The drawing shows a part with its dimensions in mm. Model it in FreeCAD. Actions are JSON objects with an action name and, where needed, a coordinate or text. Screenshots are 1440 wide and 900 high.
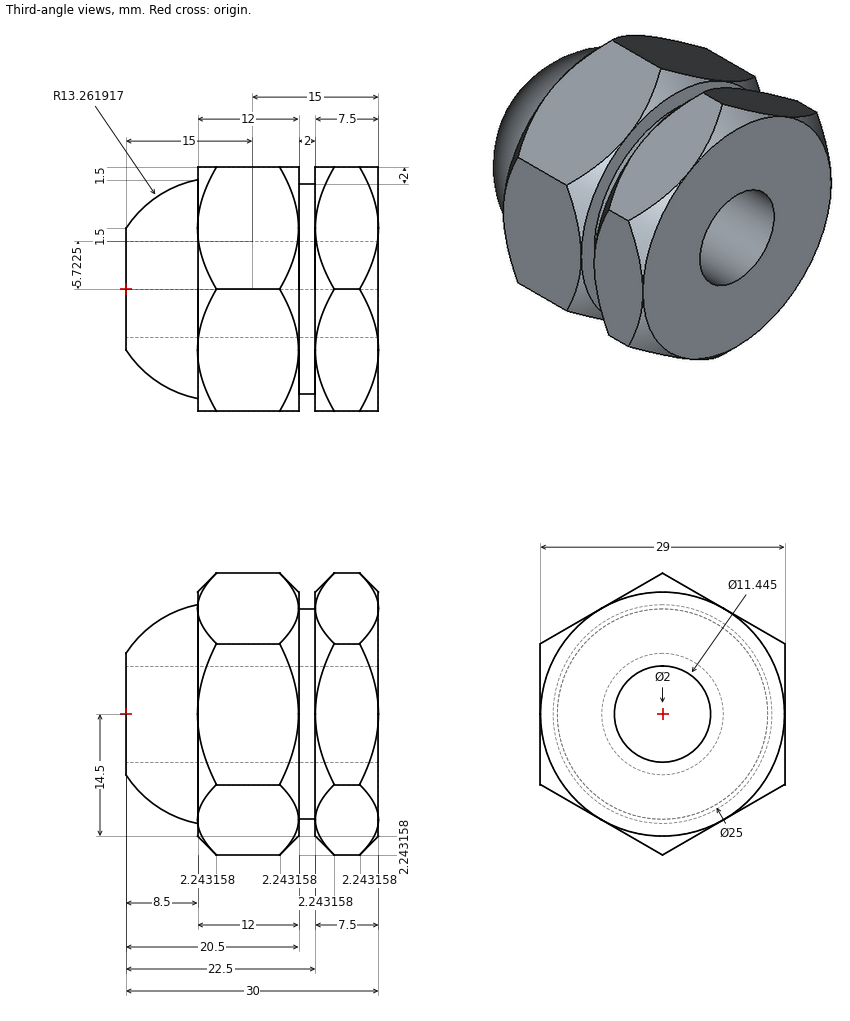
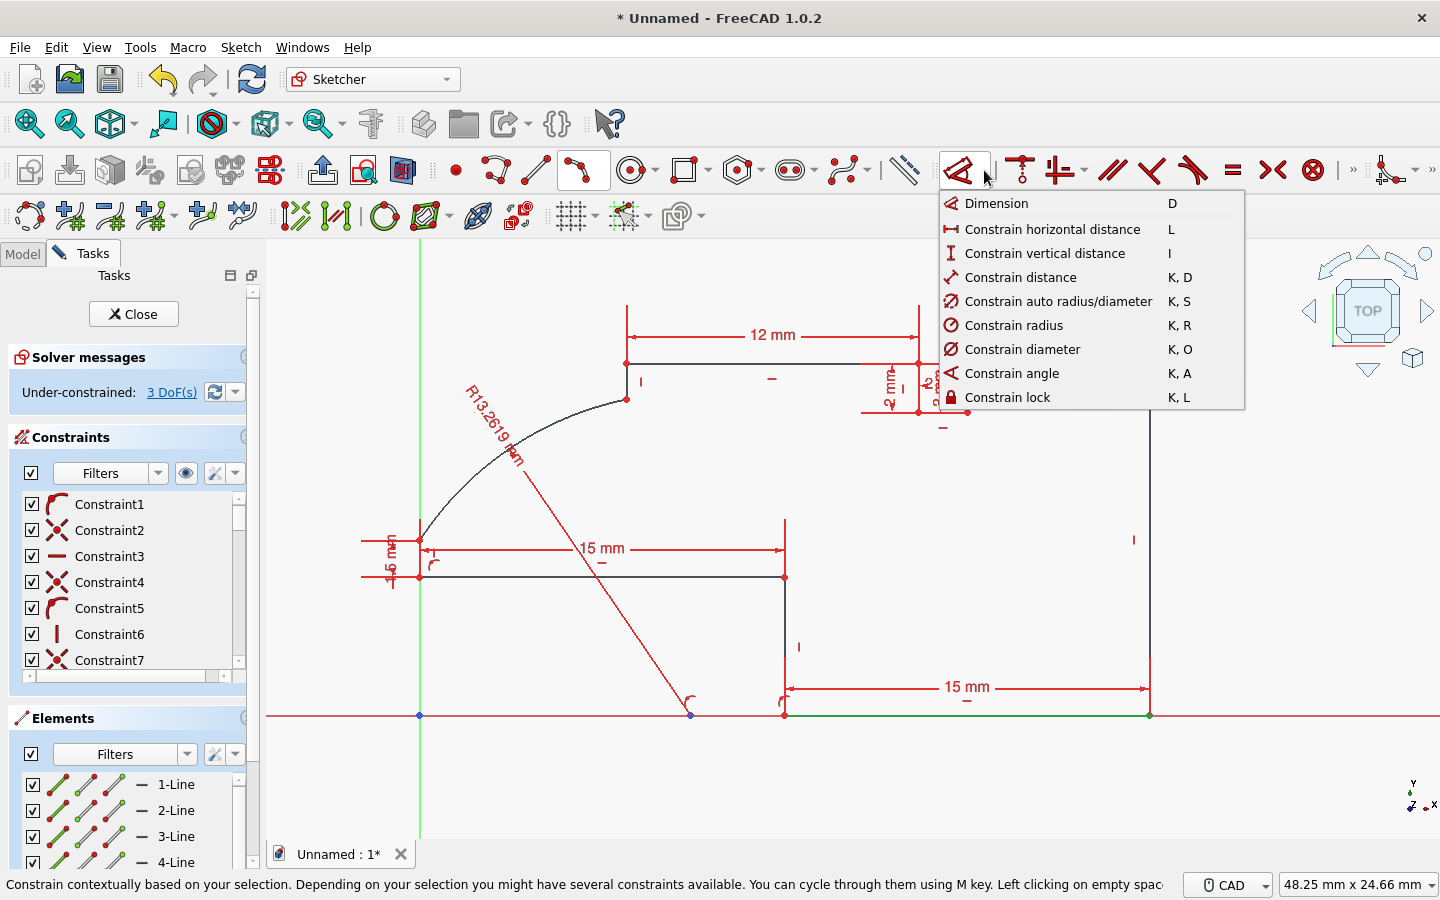
{"action": "left_click", "coordinate": [1092, 229]}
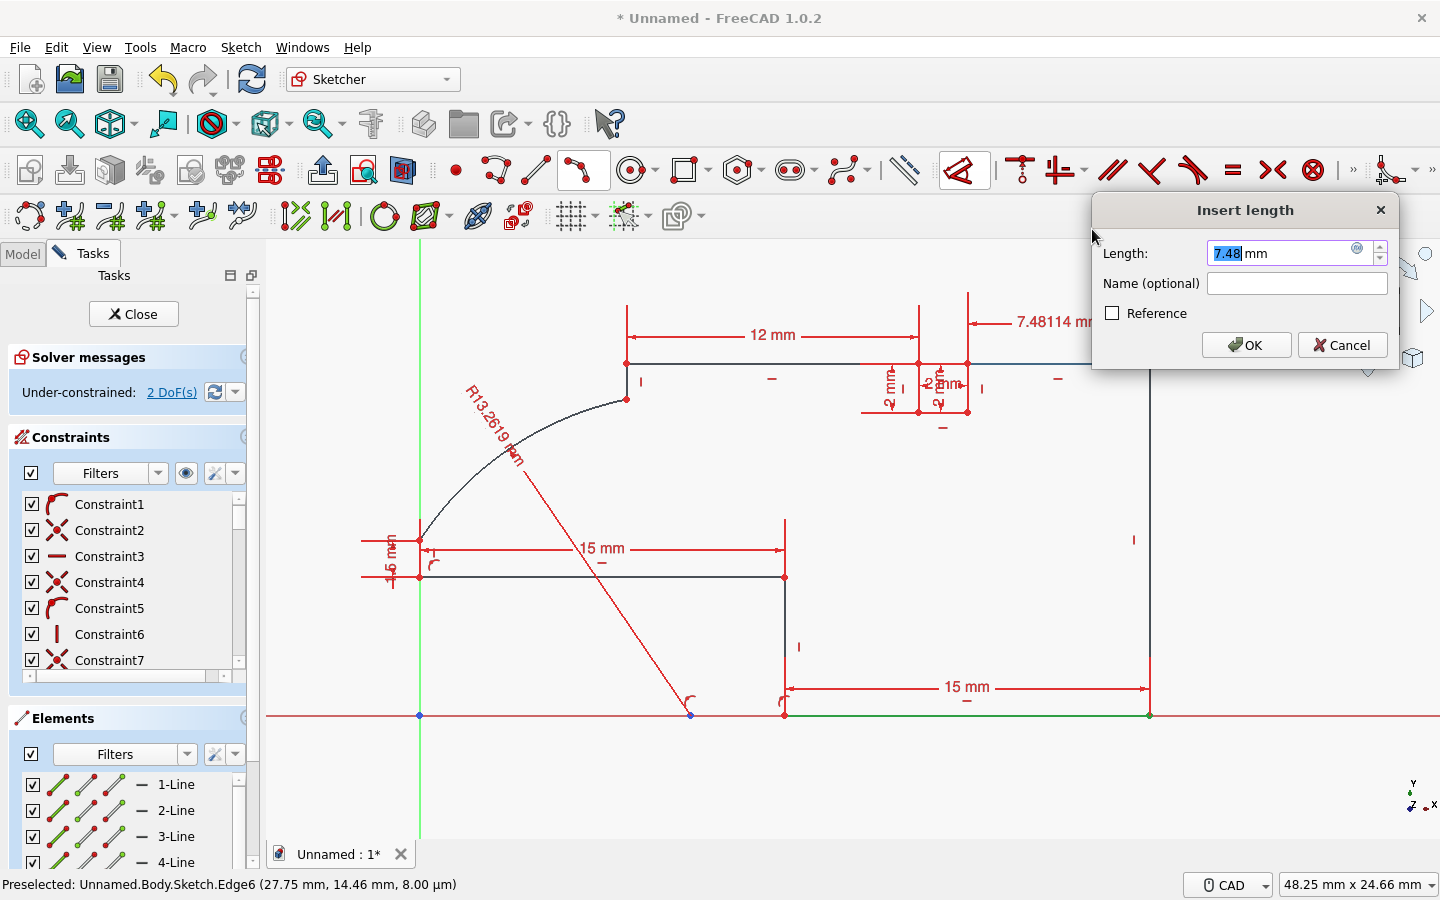
{"action": "type", "text": "7.5"}
{"action": "key", "text": "Return"}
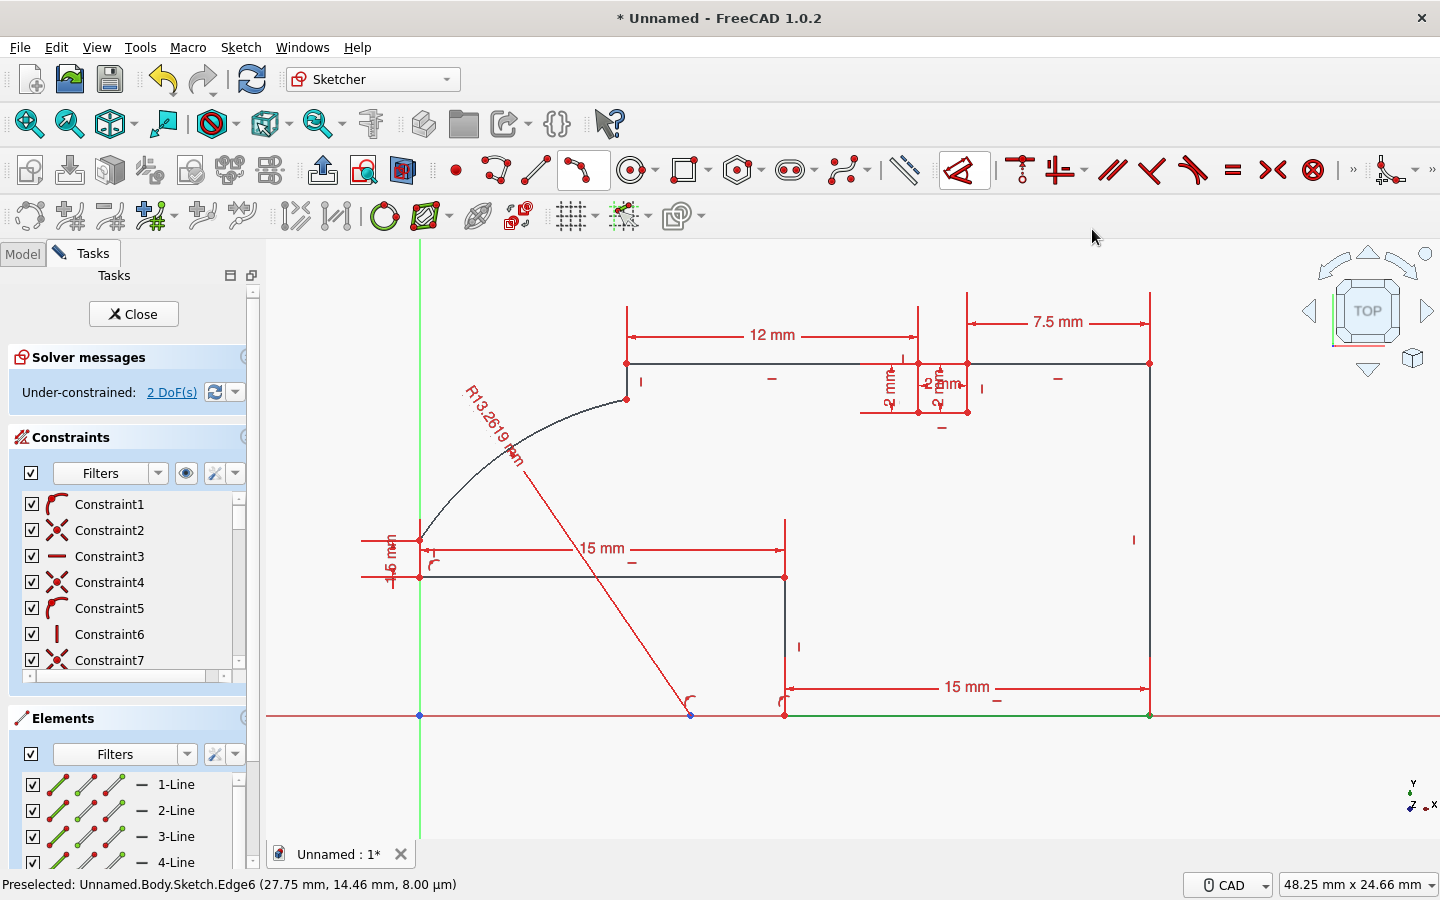
{"action": "scroll", "coordinate": [627, 375], "scroll_direction": "up", "scroll_amount": 2}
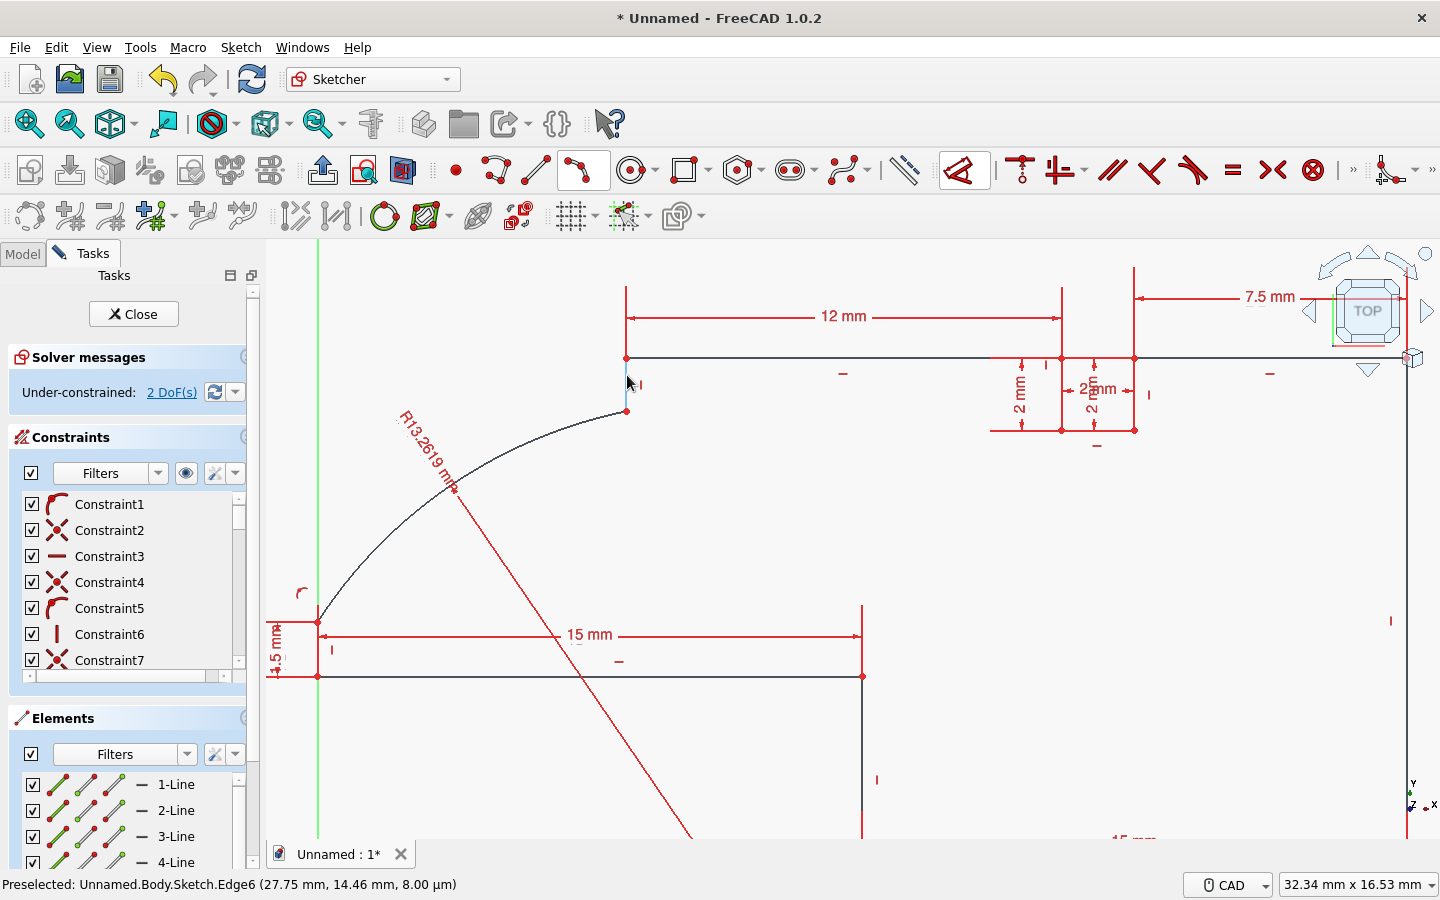
{"action": "left_click", "coordinate": [626, 374]}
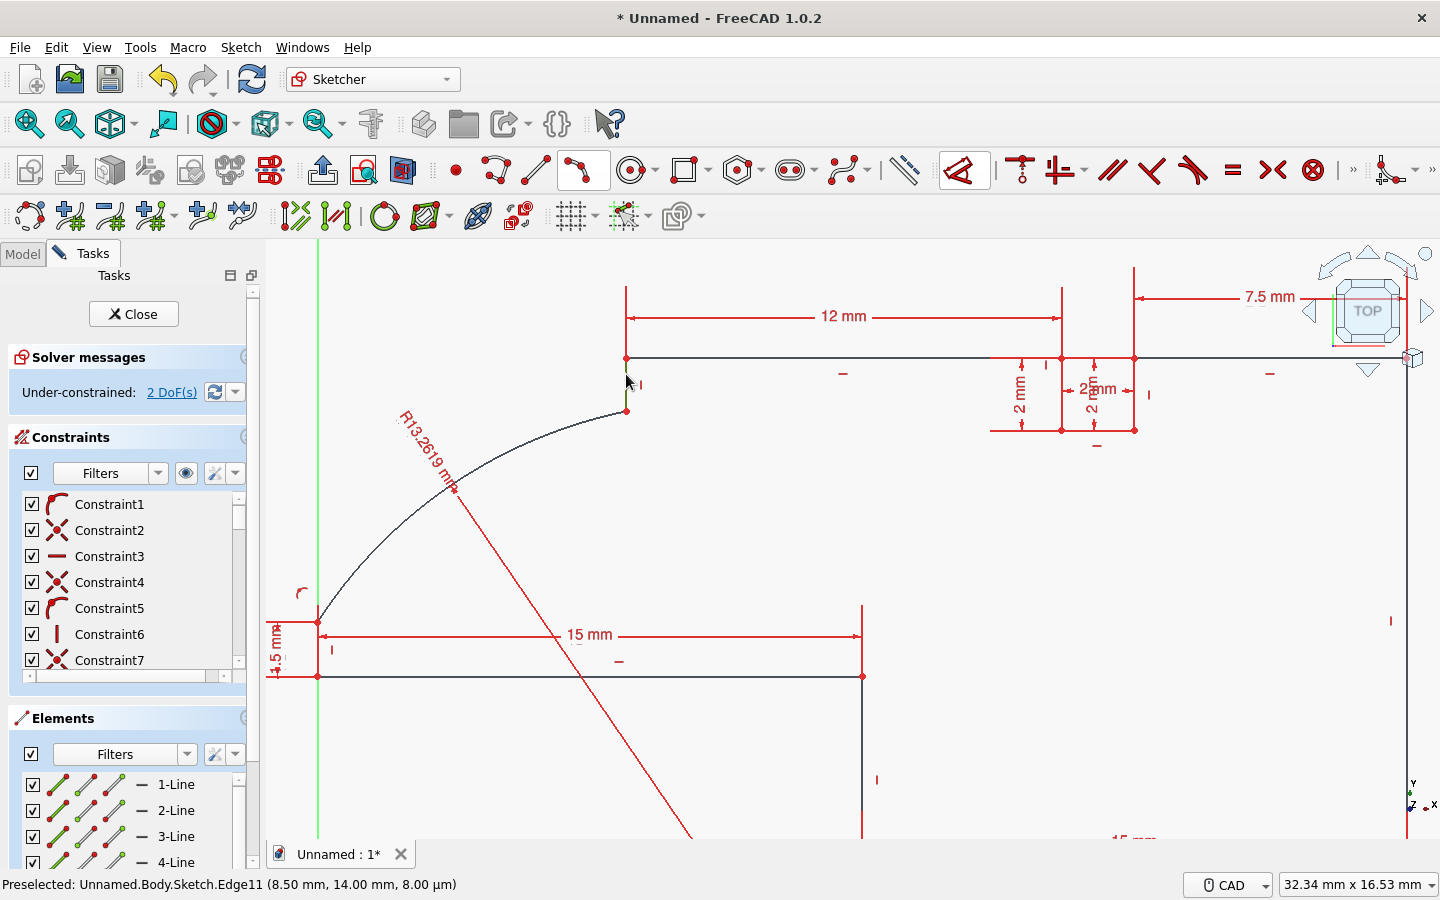
{"action": "key", "text": "i"}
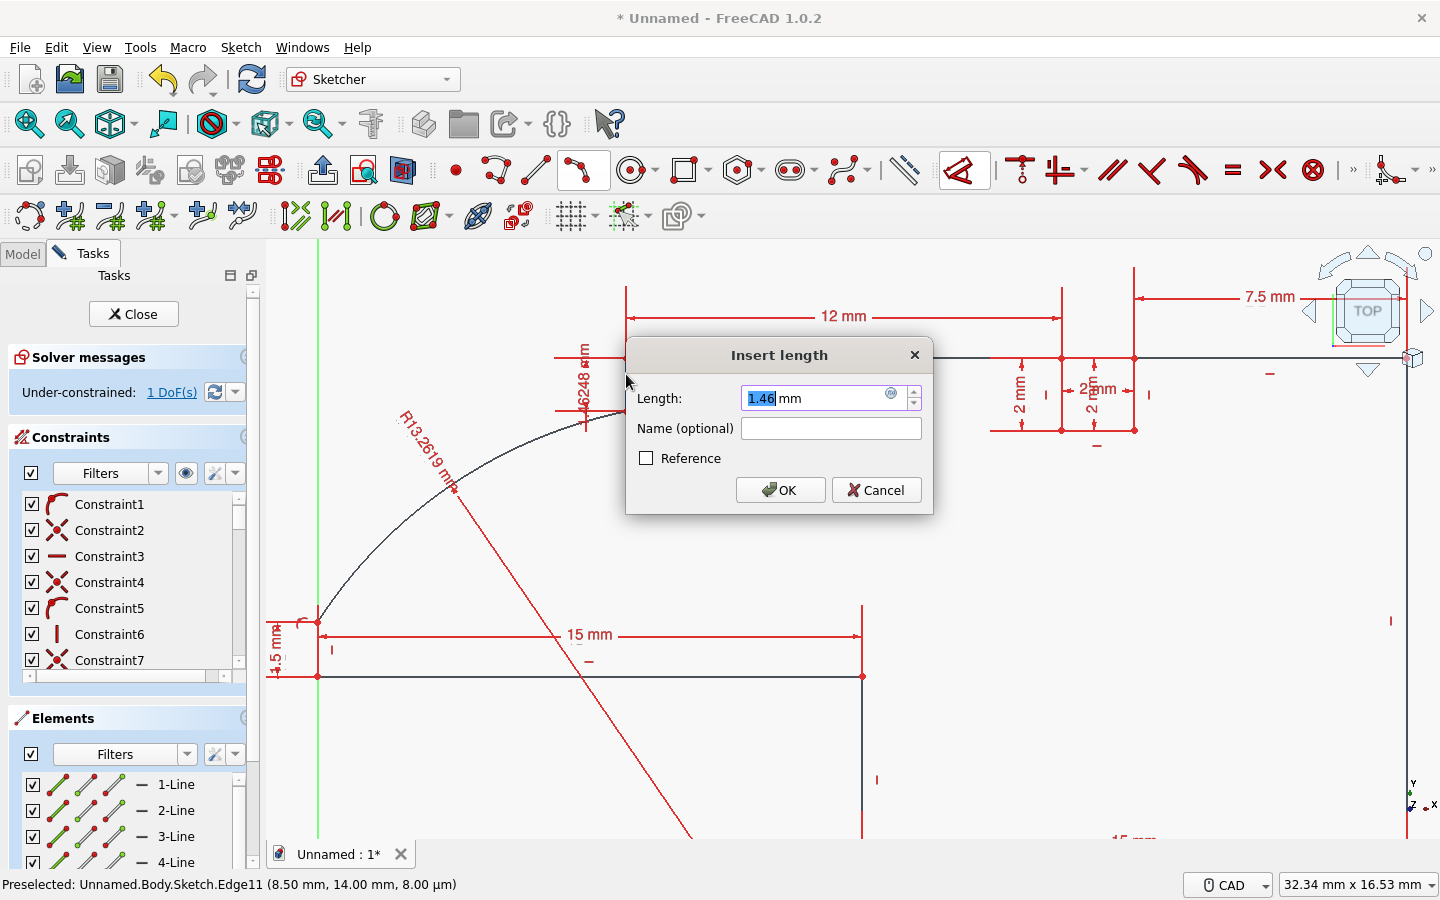
{"action": "type", "text": "1.5"}
{"action": "key", "text": "Return"}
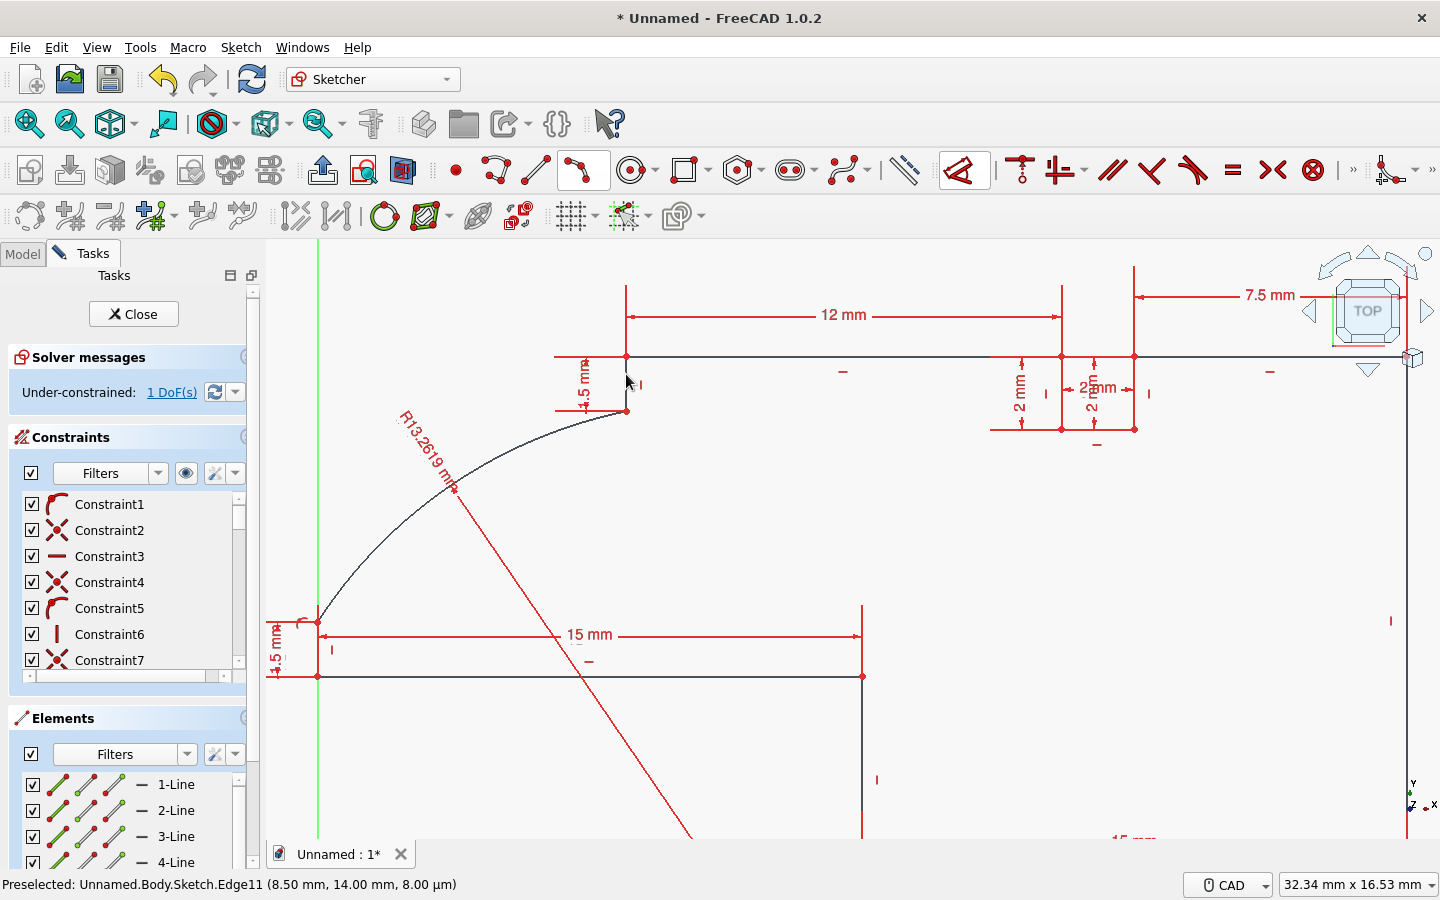
{"action": "left_click", "coordinate": [862, 739]}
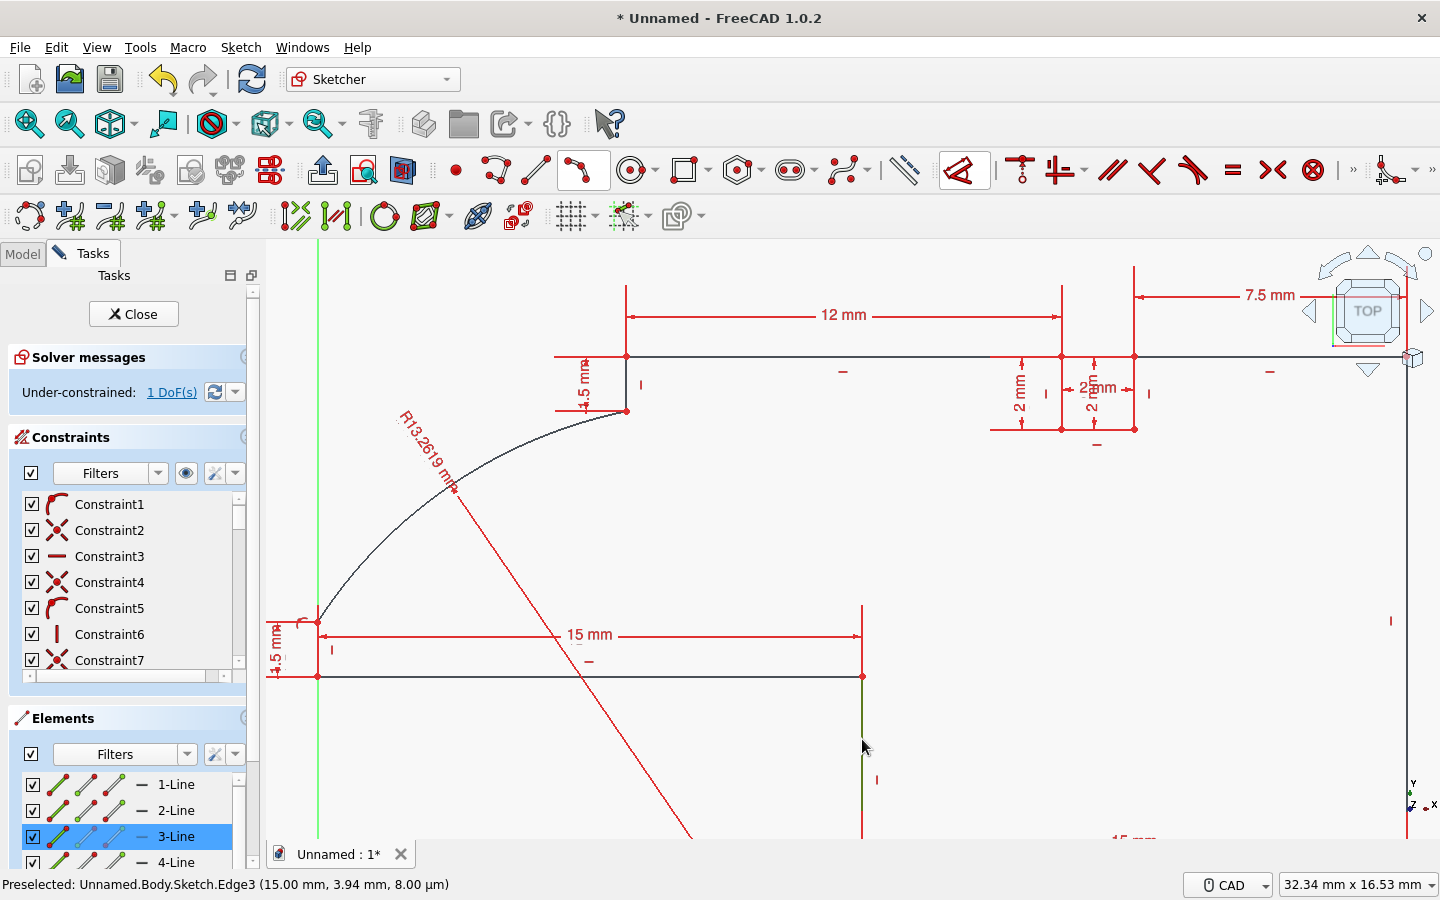
{"action": "key", "text": "i"}